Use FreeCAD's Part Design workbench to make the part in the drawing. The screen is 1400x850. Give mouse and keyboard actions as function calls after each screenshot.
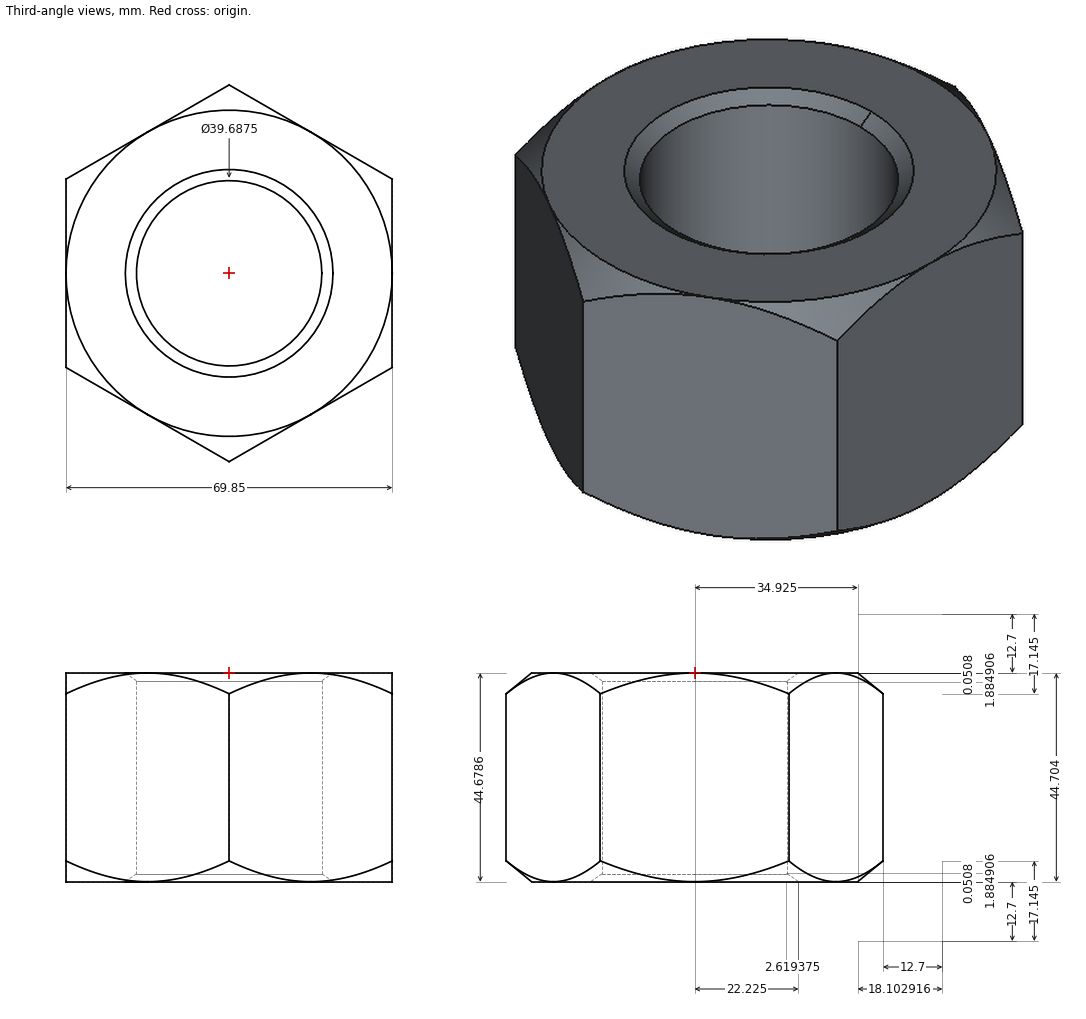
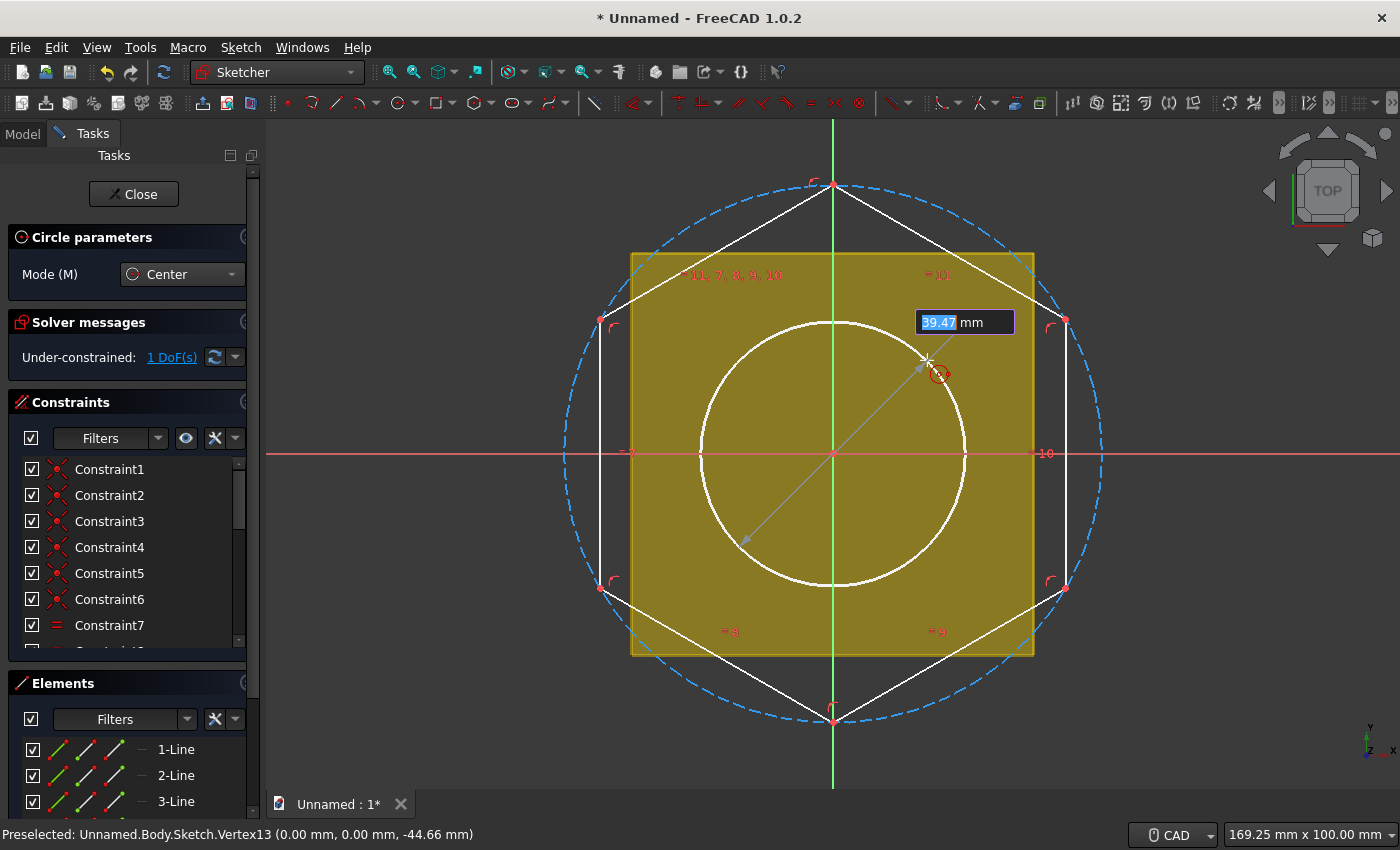
text(39.6875)
key(Return)
key(Escape)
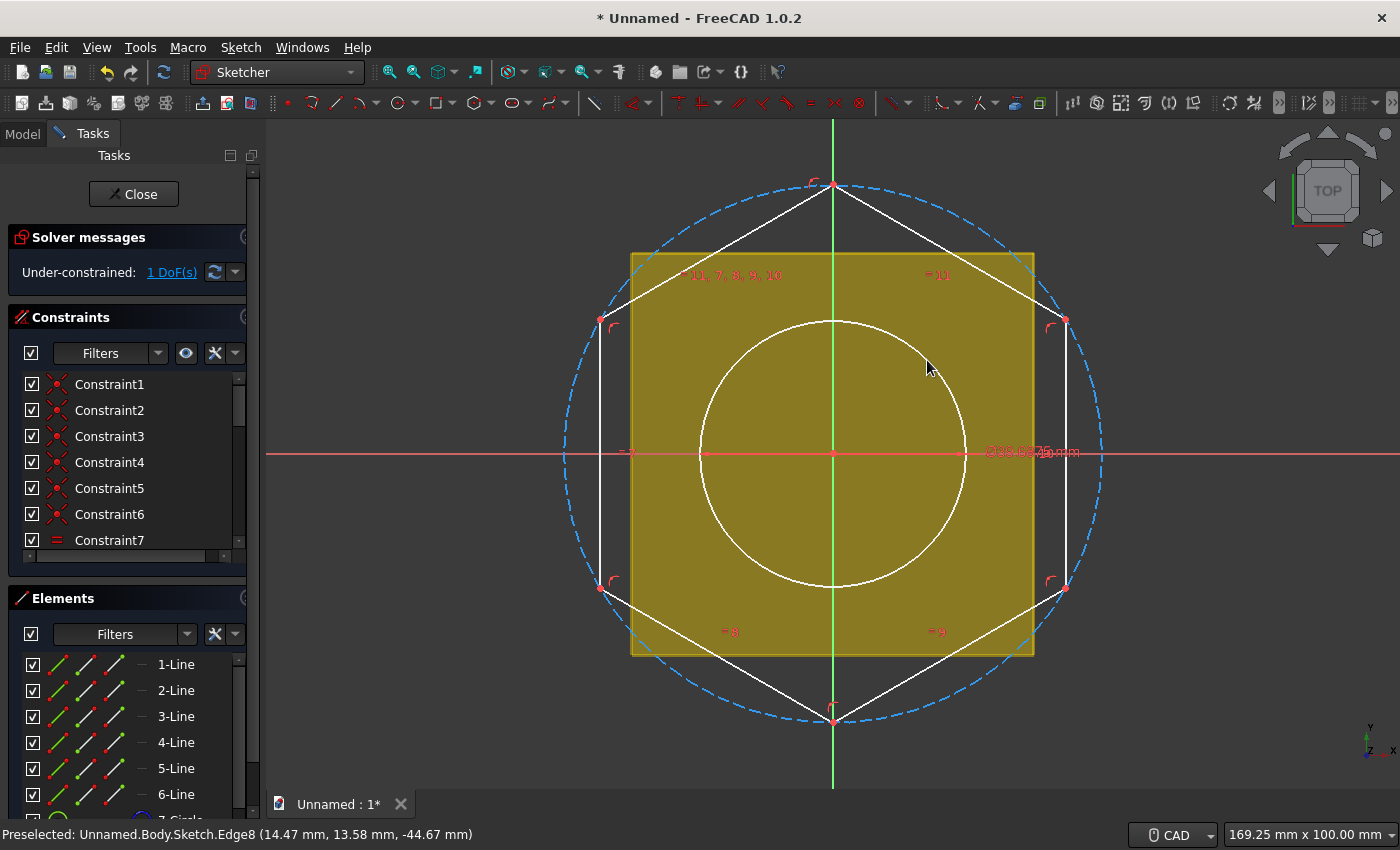
click(632, 104)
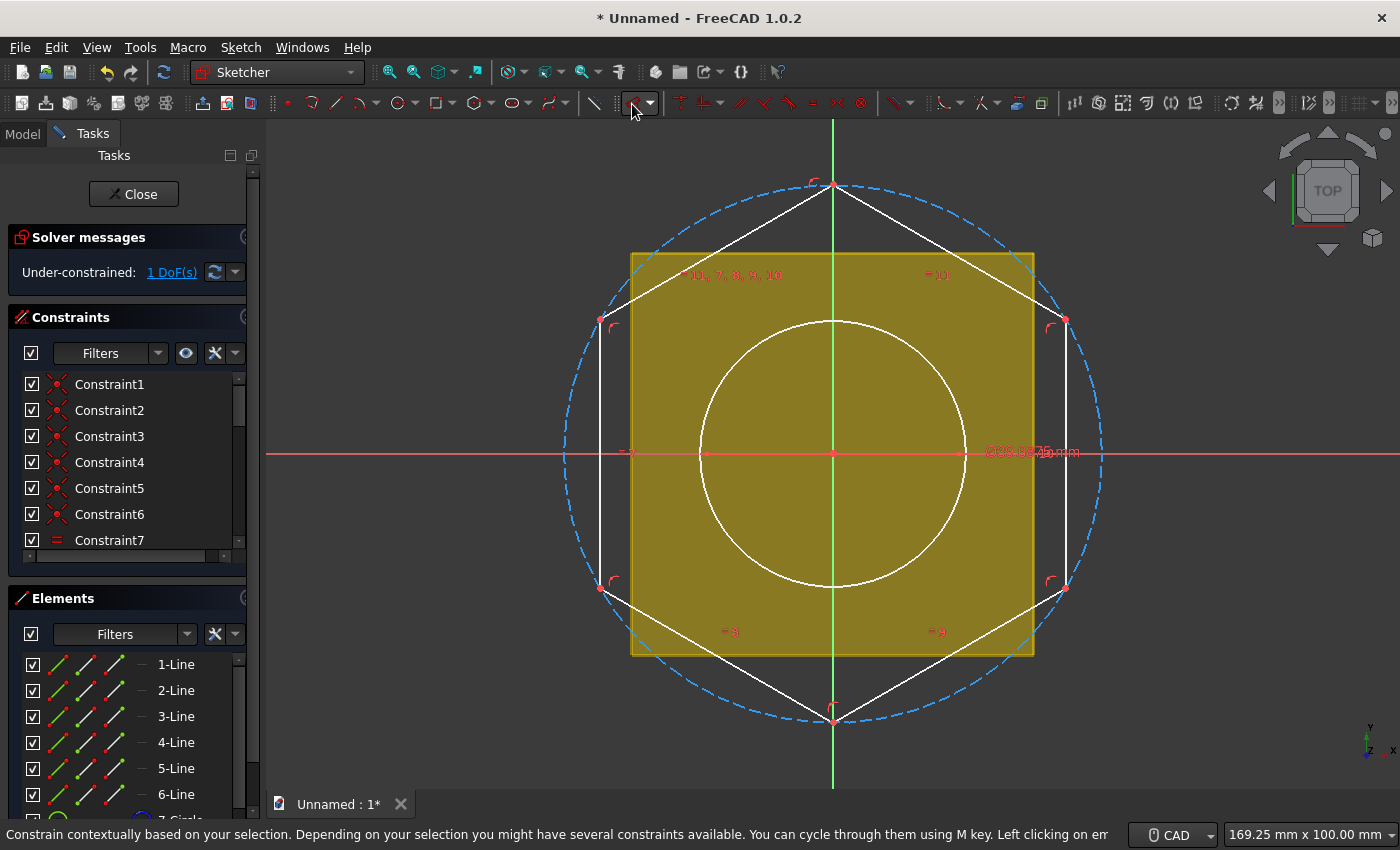
click(600, 319)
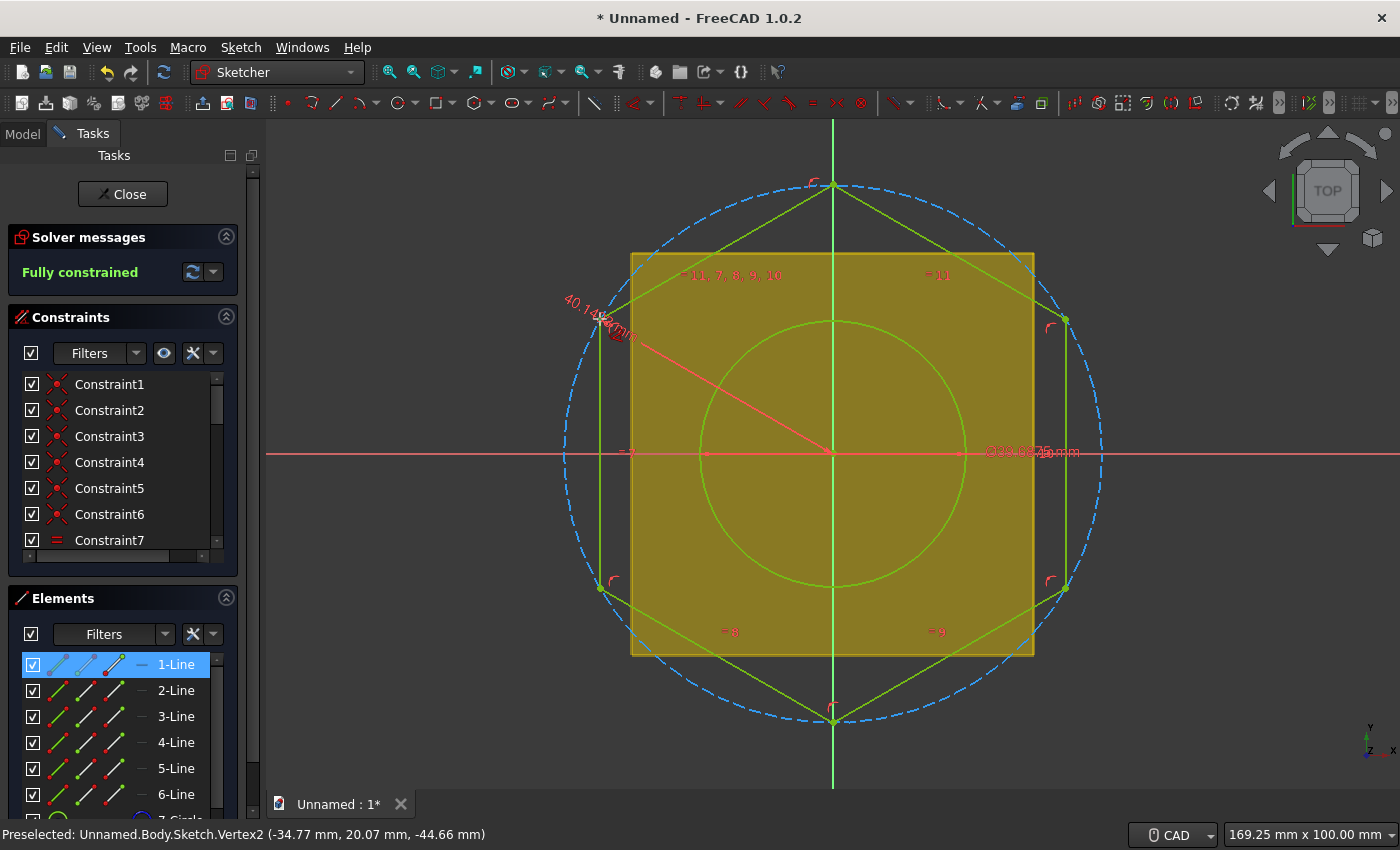
click(1066, 589)
click(726, 623)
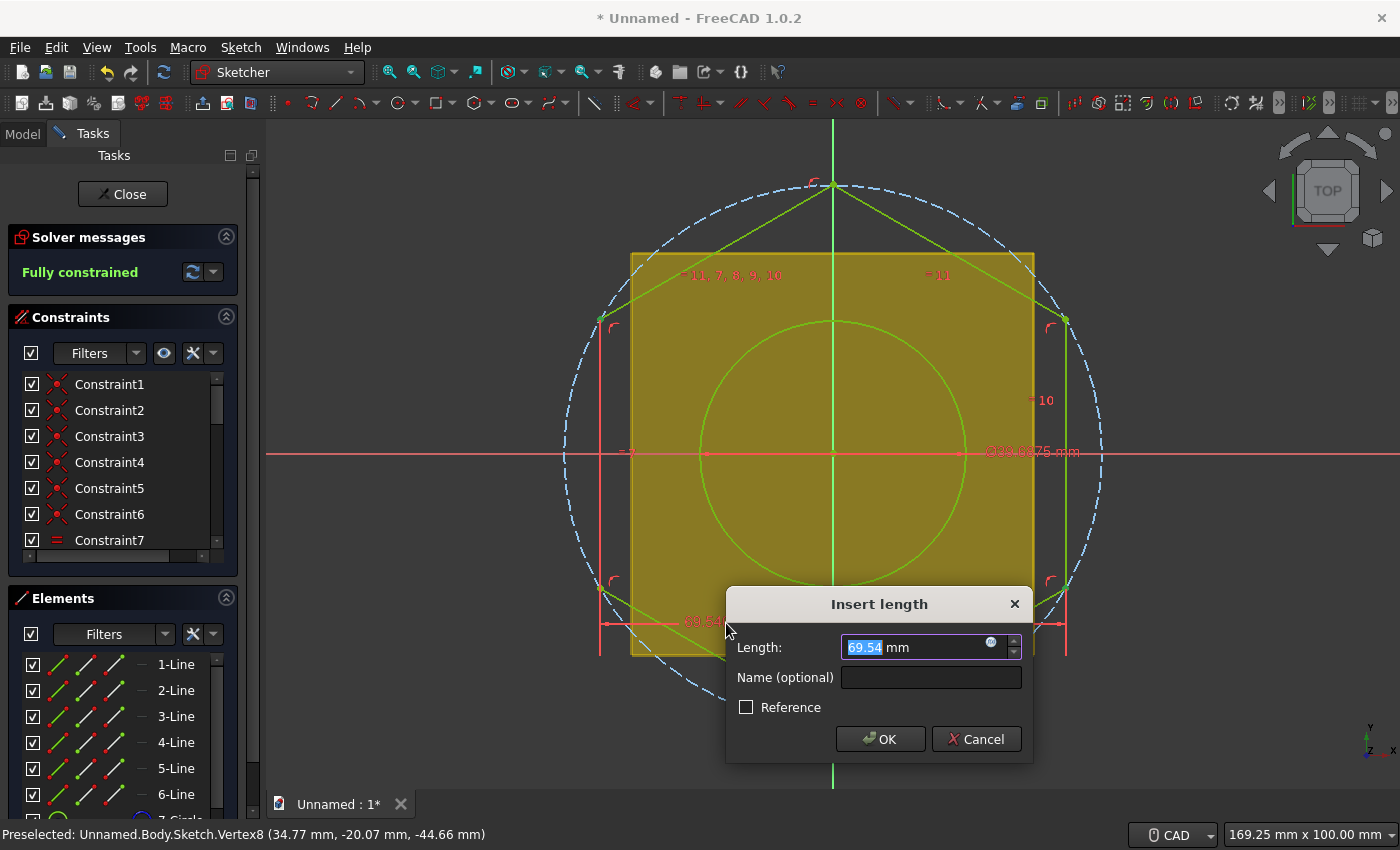
text(69.85)
key(Return)
key(Escape)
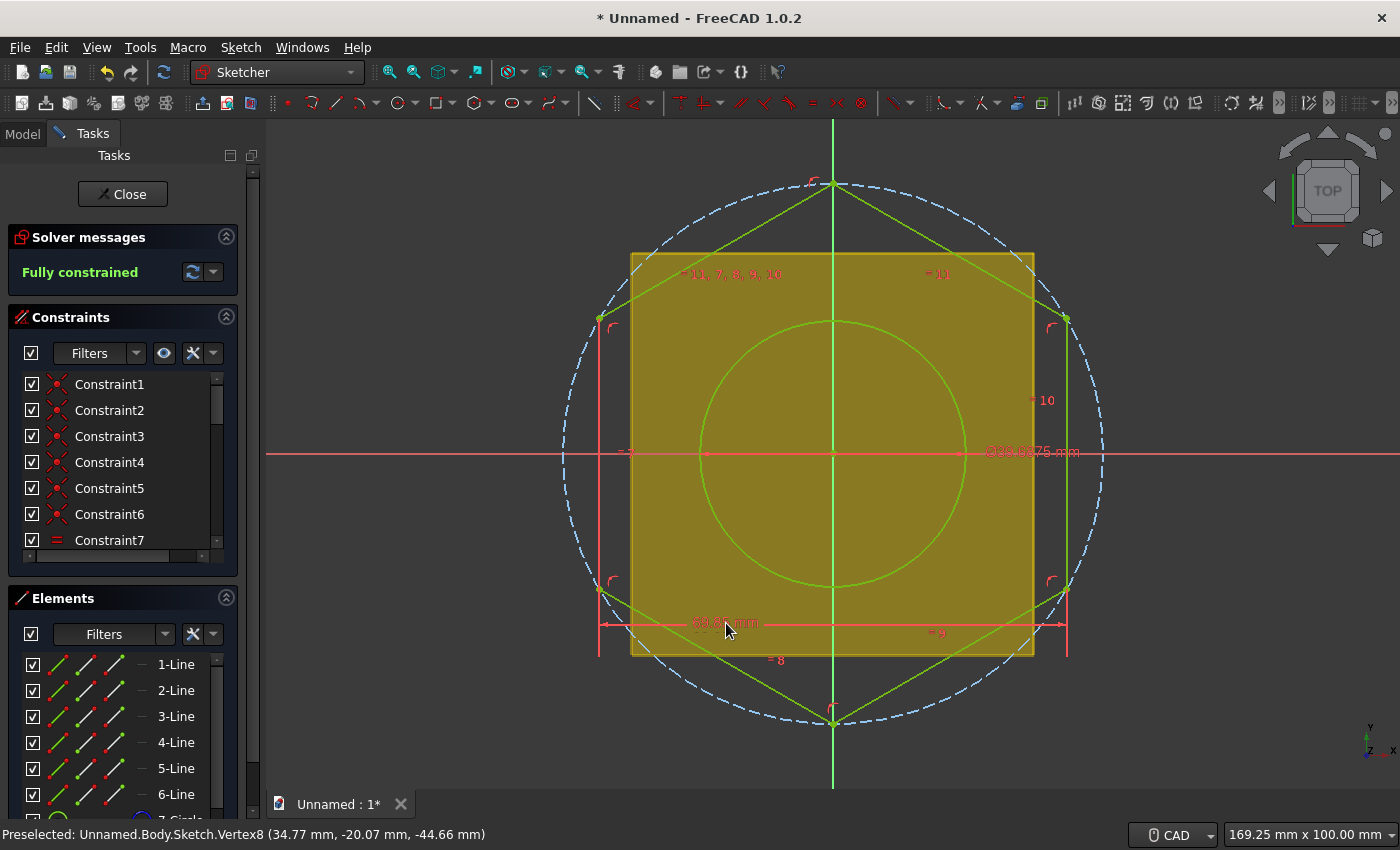
click(123, 194)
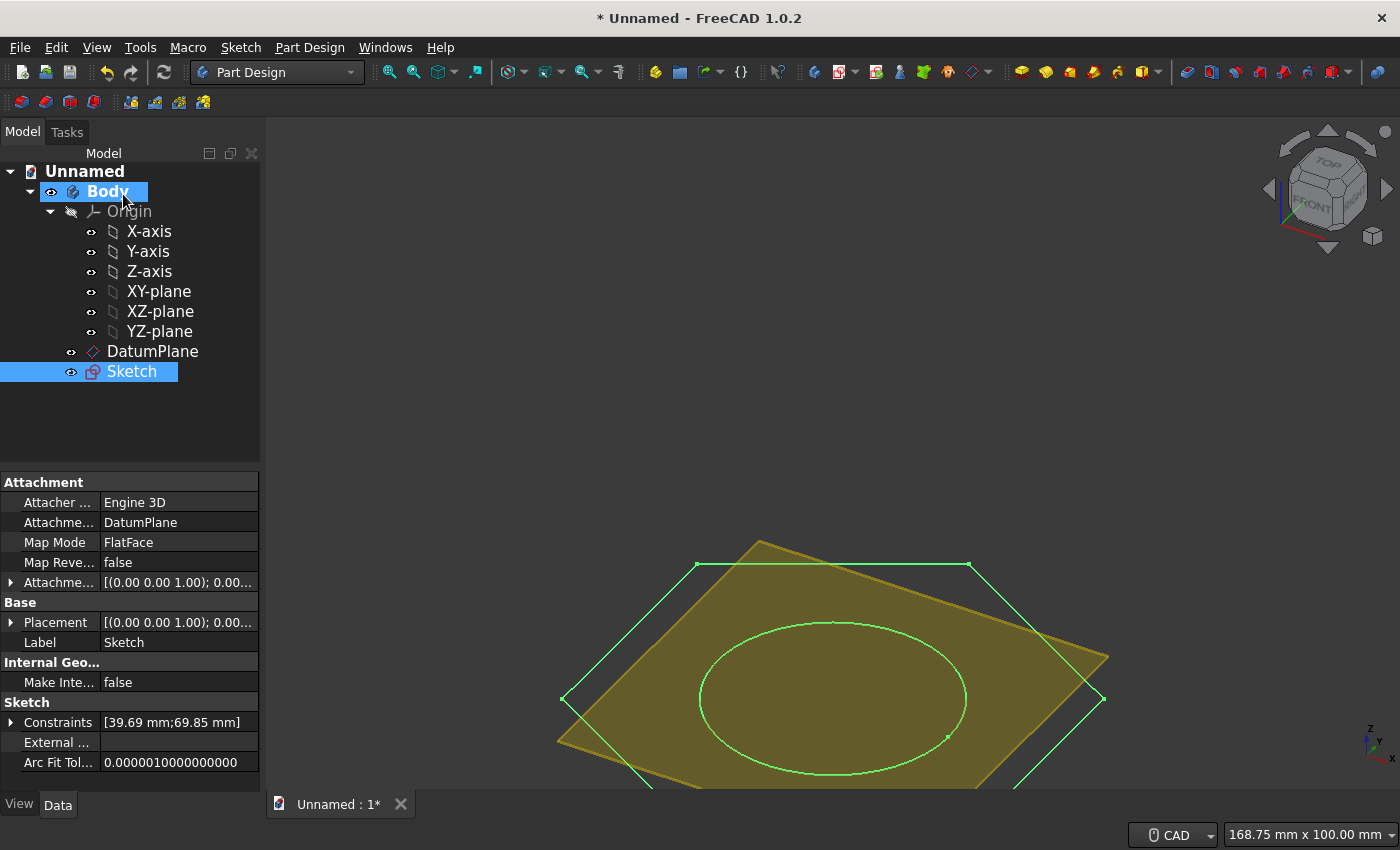
click(1022, 72)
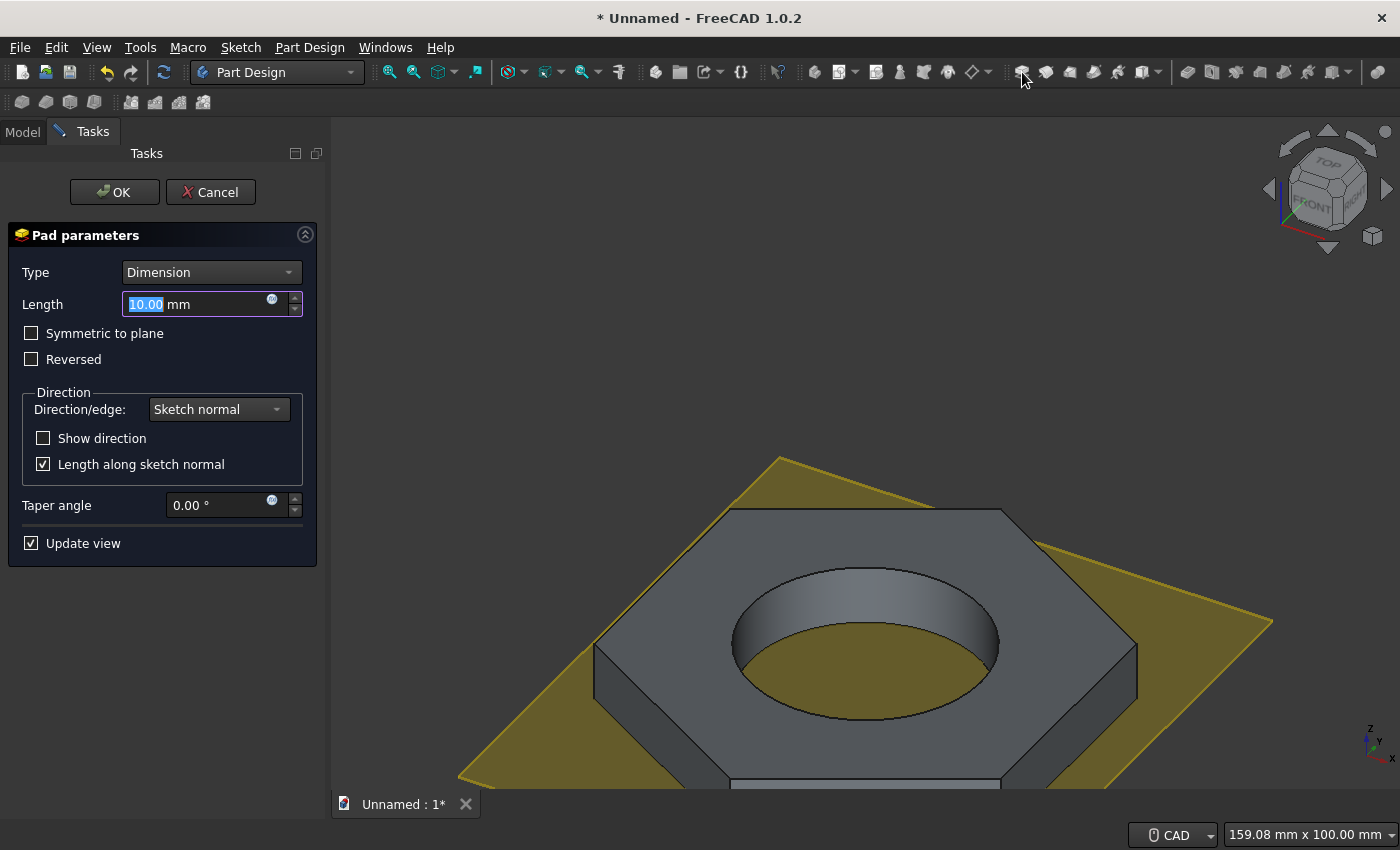
text(44.6786)
key(Tab)